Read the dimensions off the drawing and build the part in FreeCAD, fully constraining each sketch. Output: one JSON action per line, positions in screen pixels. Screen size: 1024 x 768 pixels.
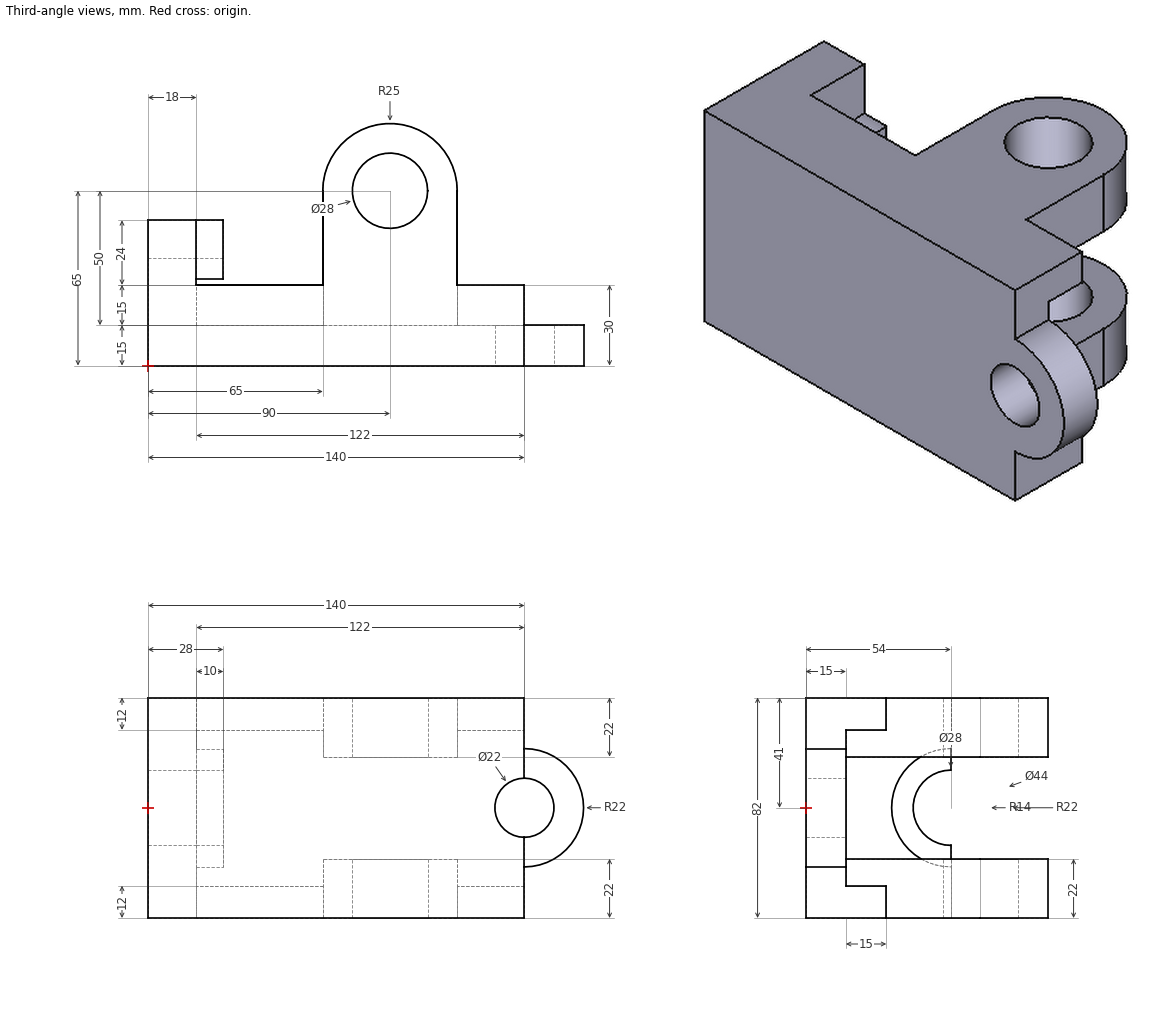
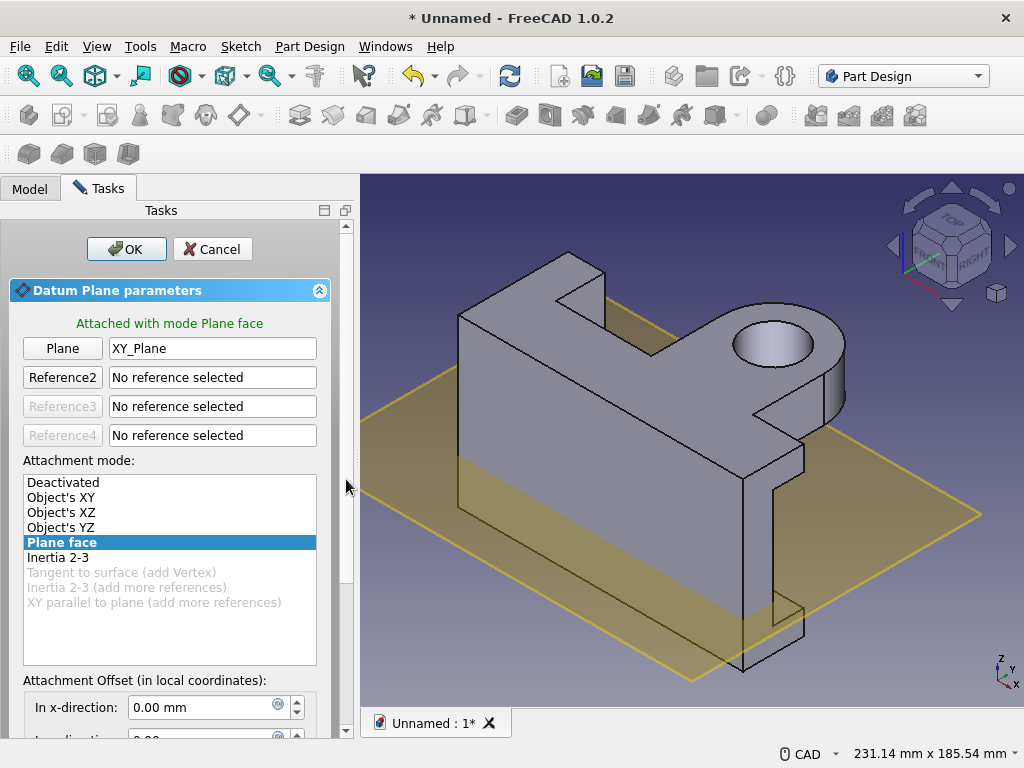
{"action": "left_click", "coordinate": [127, 249]}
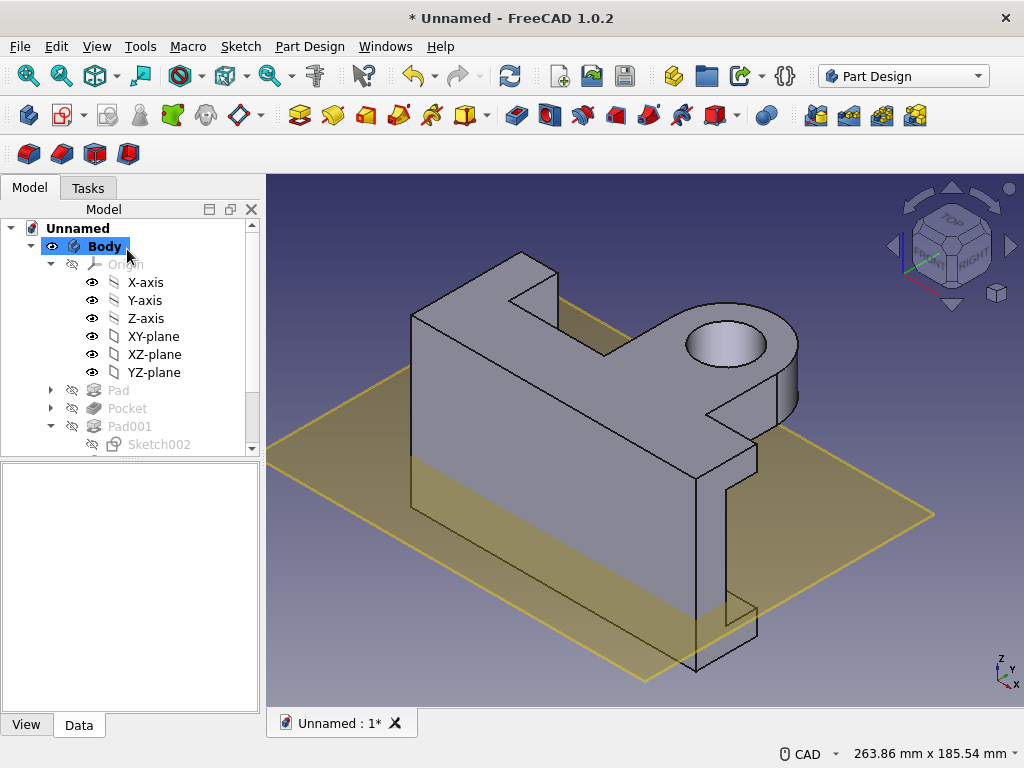
{"action": "scroll", "coordinate": [101, 332], "scroll_direction": "down", "scroll_amount": 3}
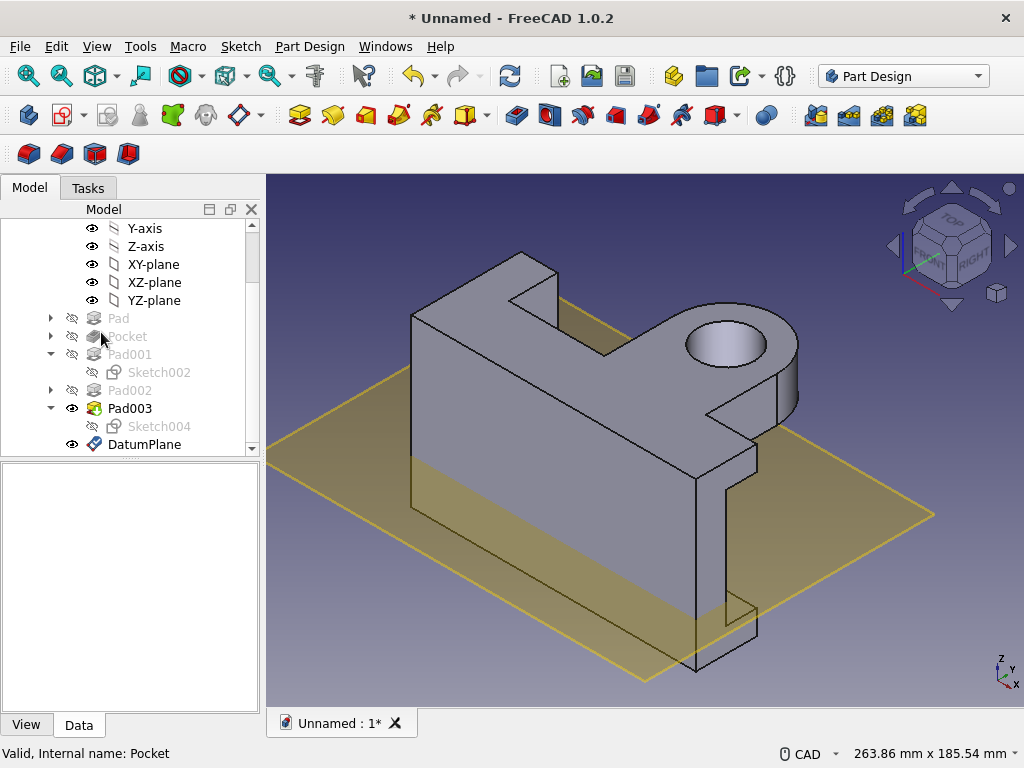
{"action": "left_click", "coordinate": [117, 444]}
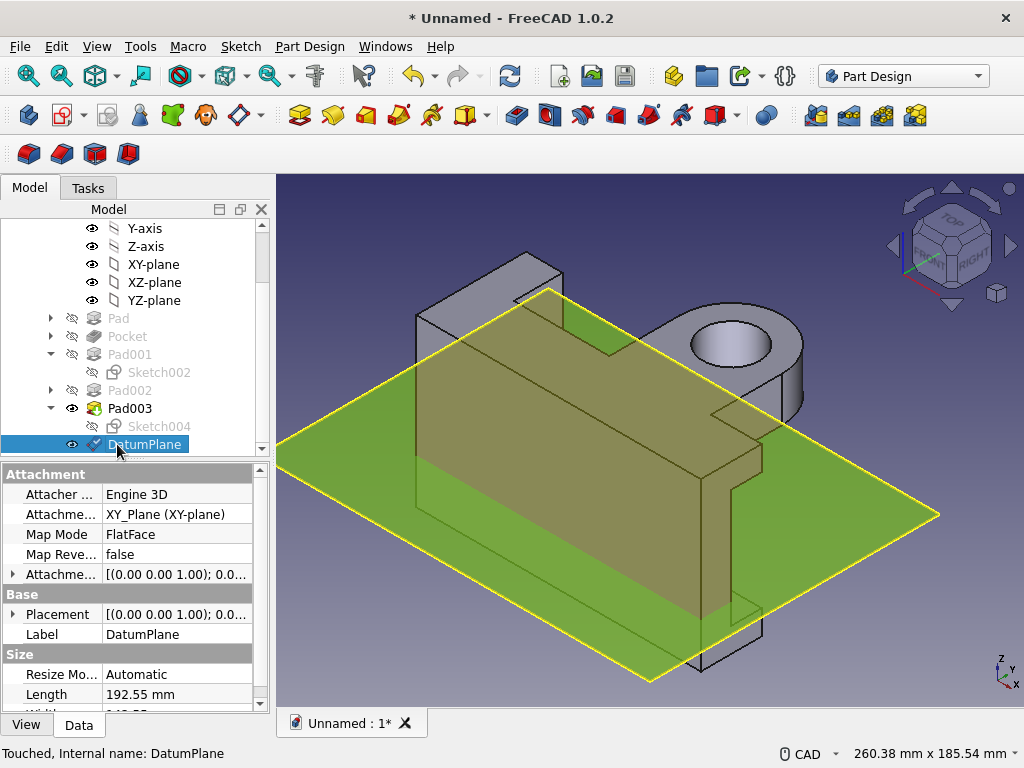
{"action": "left_click", "coordinate": [62, 116]}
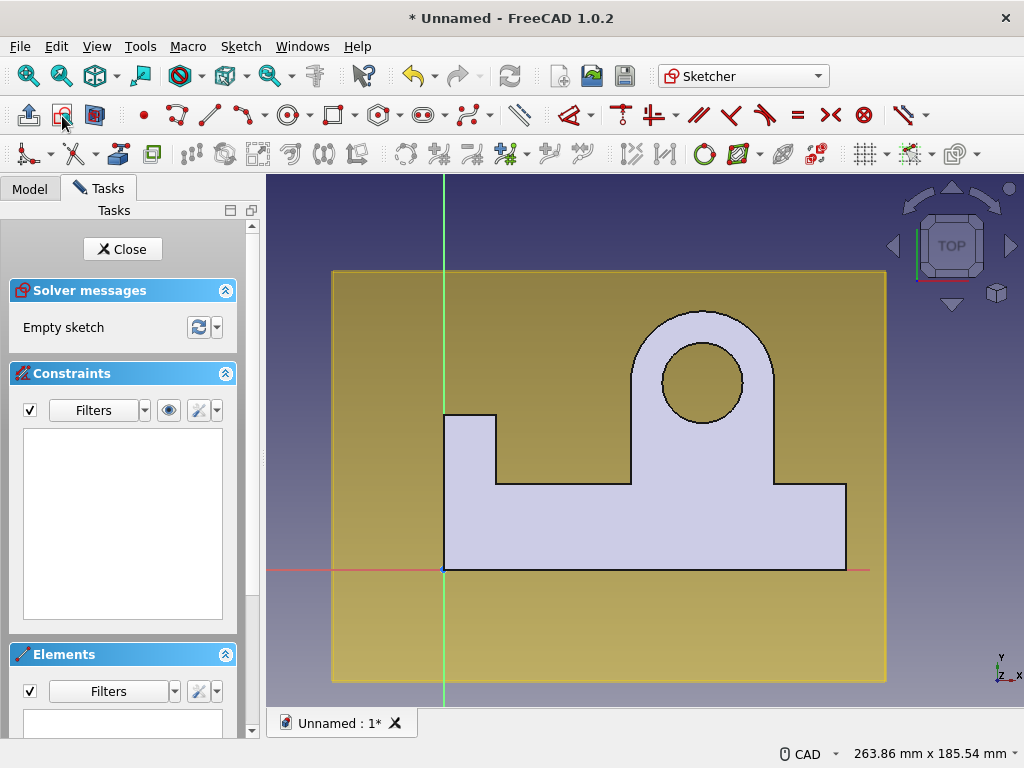
{"action": "key", "text": "q s"}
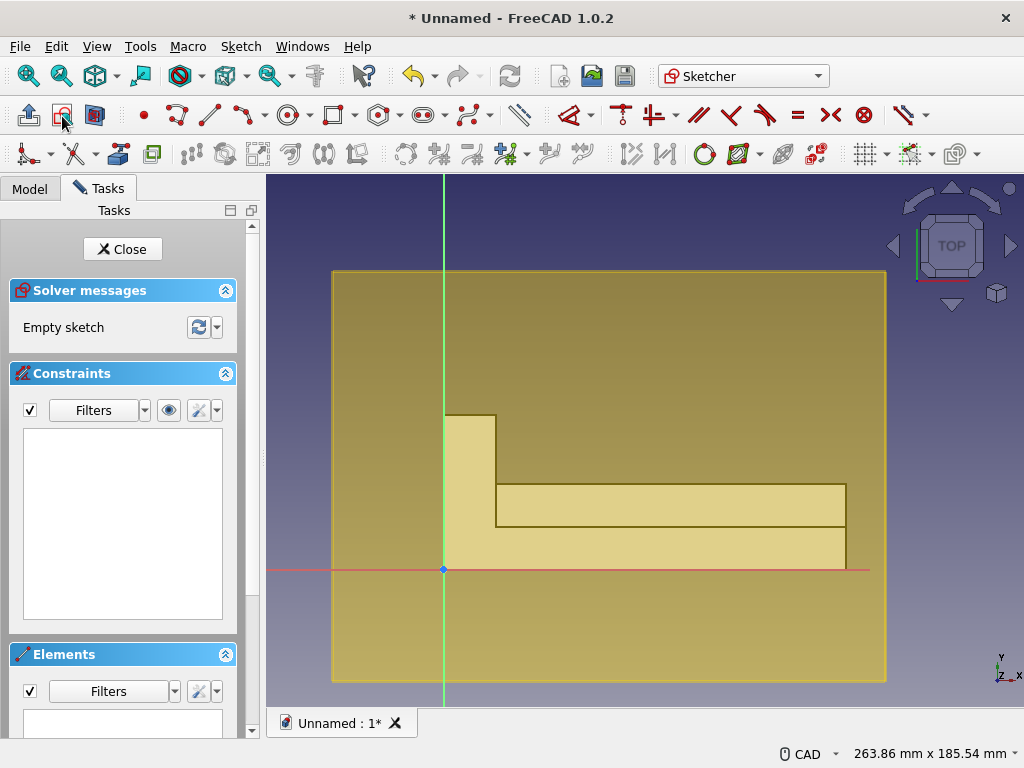
{"action": "left_click", "coordinate": [177, 116]}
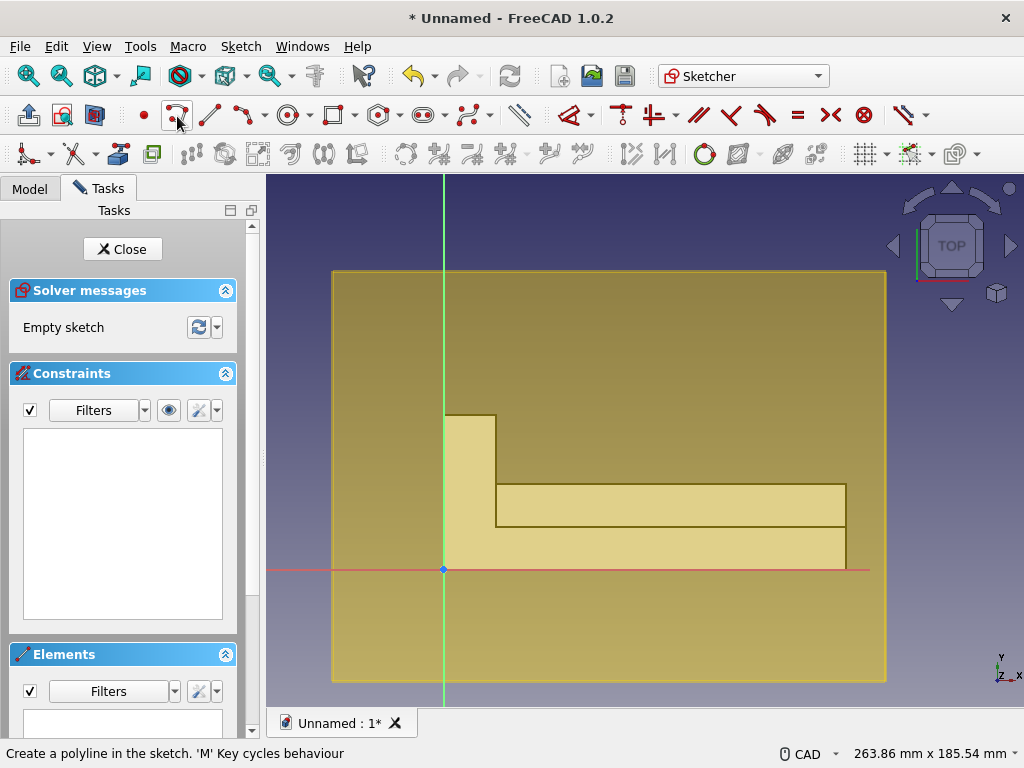
{"action": "left_click", "coordinate": [774, 383]}
{"action": "left_click", "coordinate": [774, 527]}
{"action": "left_click", "coordinate": [631, 527]}
{"action": "left_click", "coordinate": [631, 383]}
{"action": "right_click", "coordinate": [631, 383]}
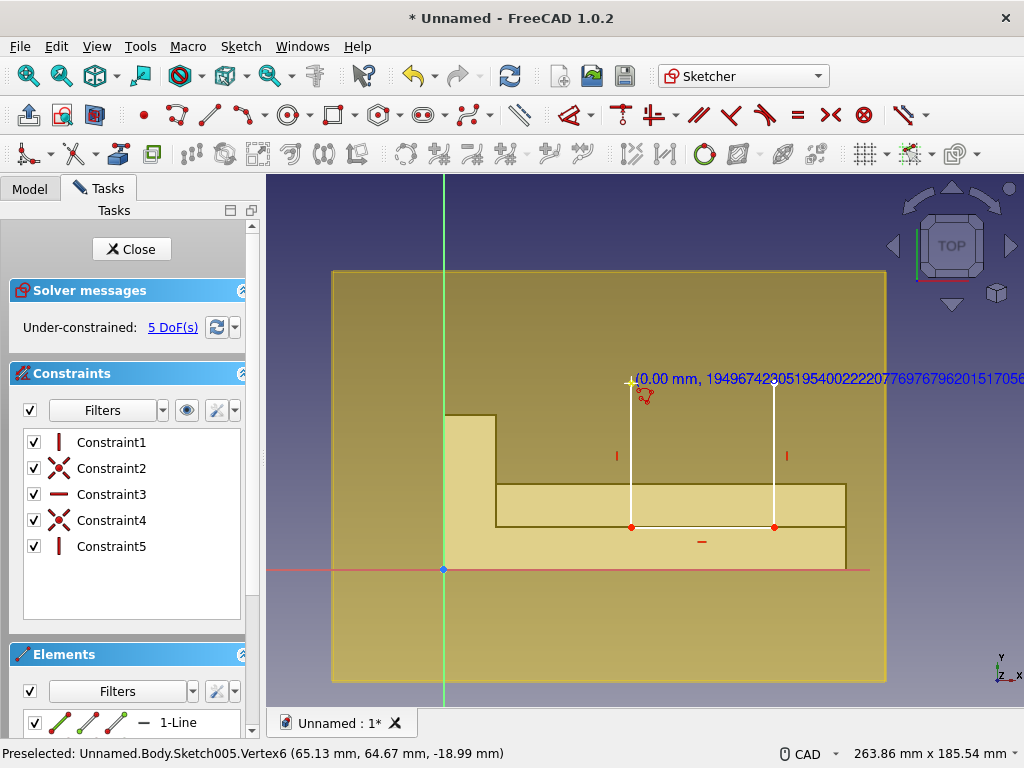
{"action": "key", "text": "g 3 a"}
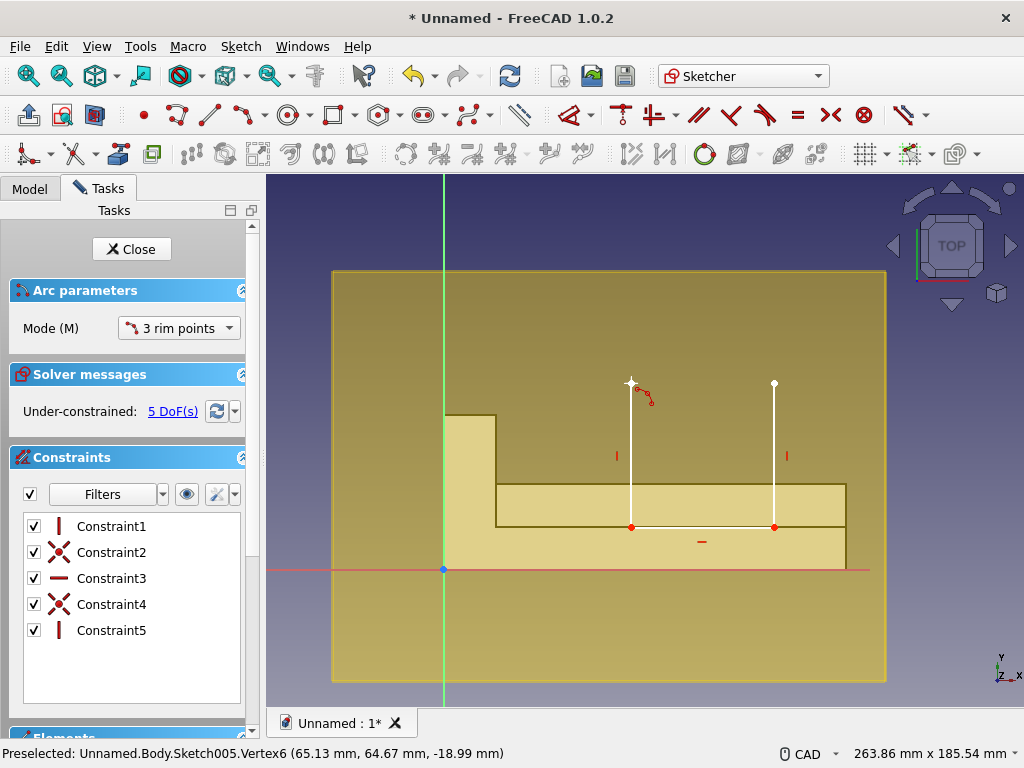
{"action": "left_click", "coordinate": [631, 384]}
{"action": "left_click", "coordinate": [774, 384]}
{"action": "left_click", "coordinate": [702, 311]}
{"action": "key", "text": "Escape"}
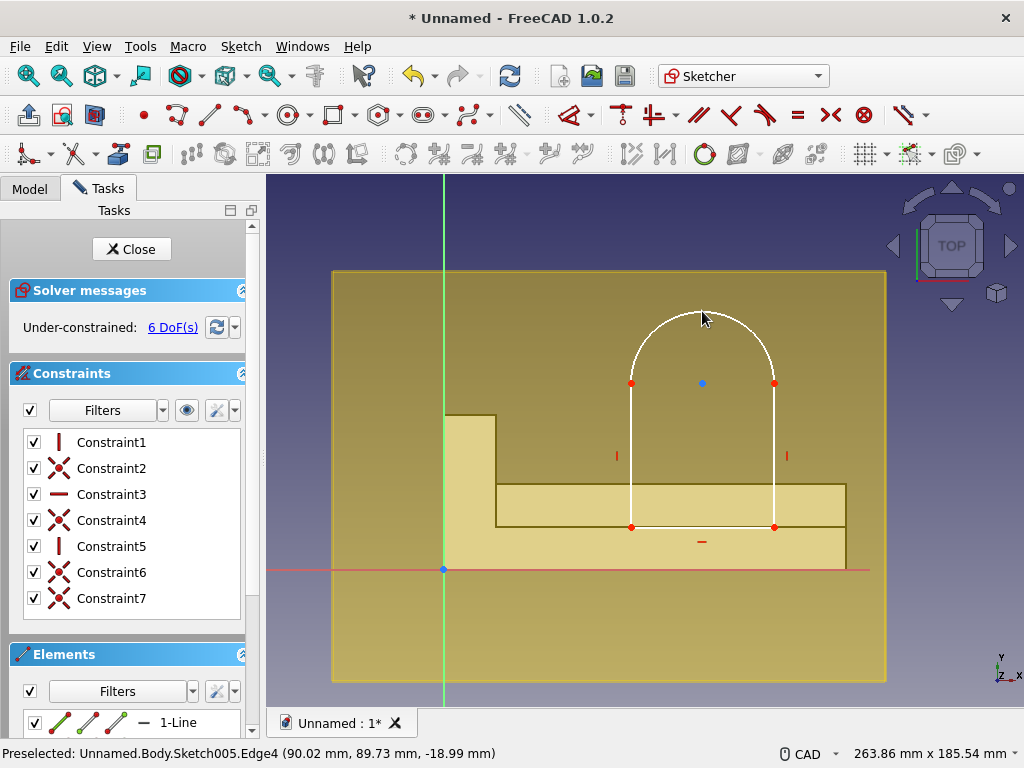
{"action": "left_click", "coordinate": [774, 427]}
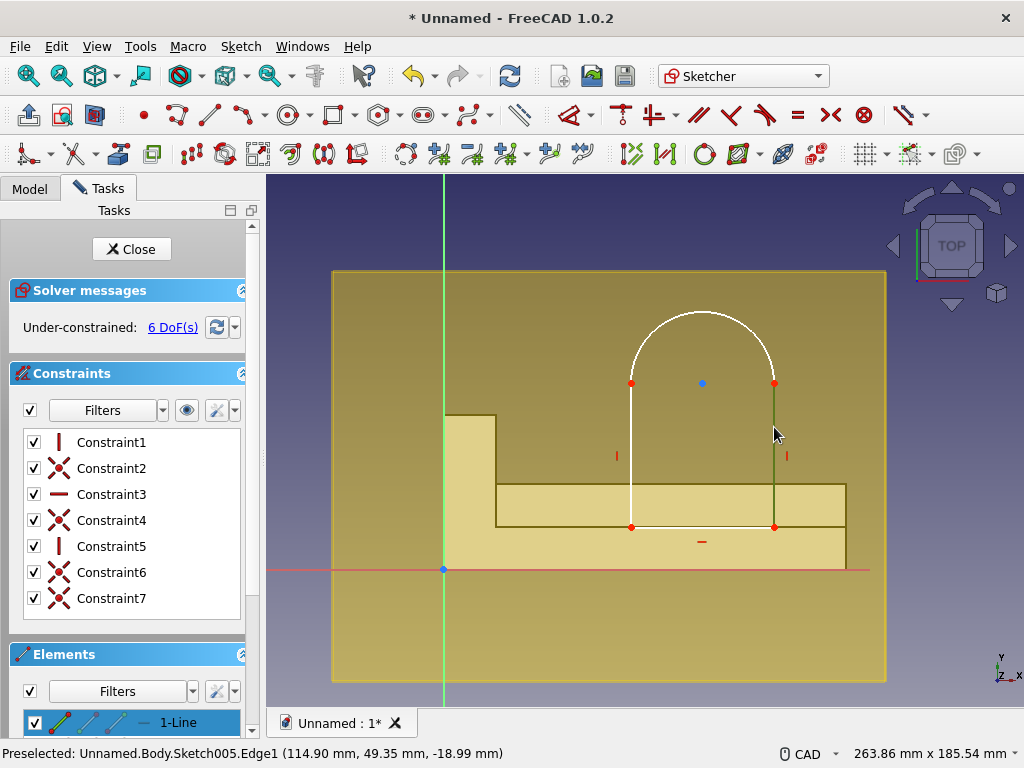
{"action": "left_click", "coordinate": [745, 326]}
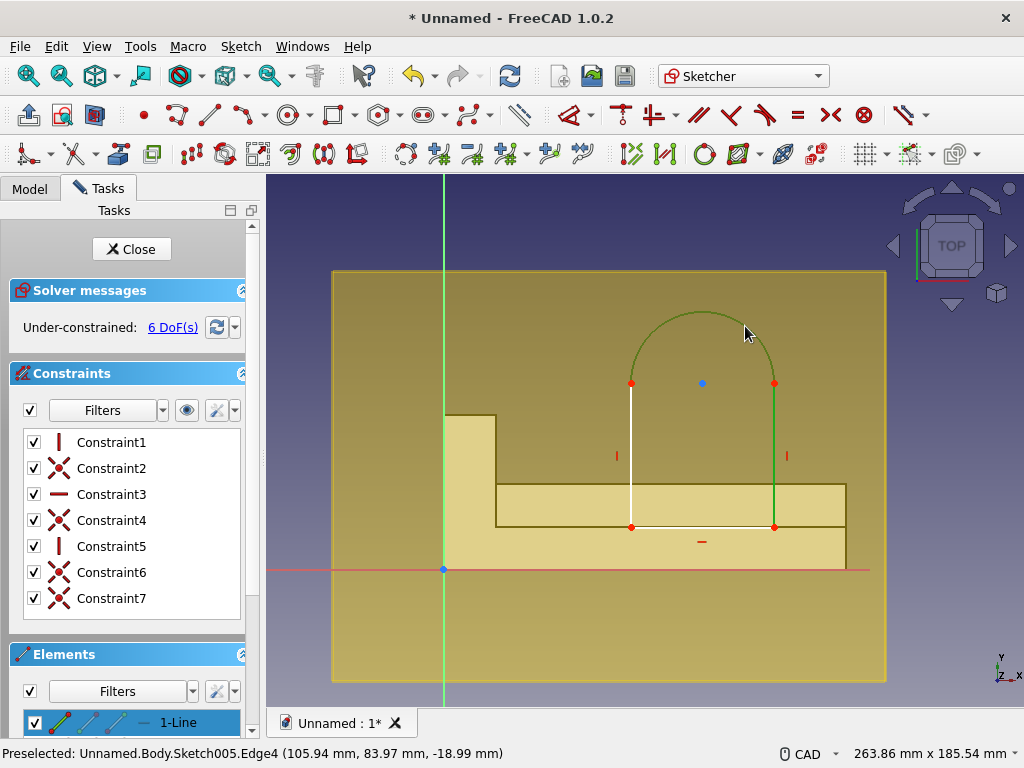
{"action": "key", "text": "t"}